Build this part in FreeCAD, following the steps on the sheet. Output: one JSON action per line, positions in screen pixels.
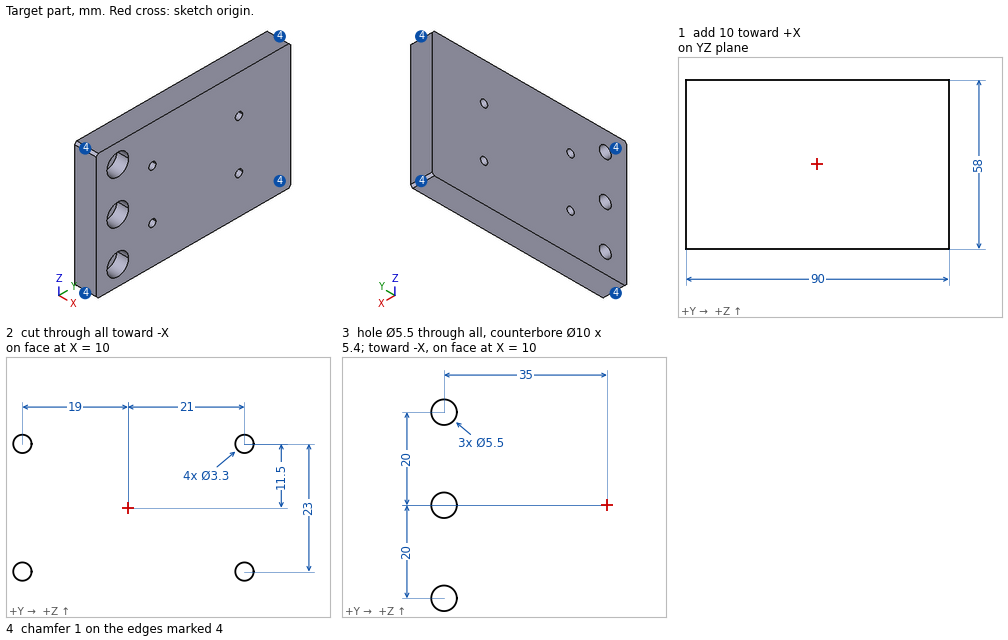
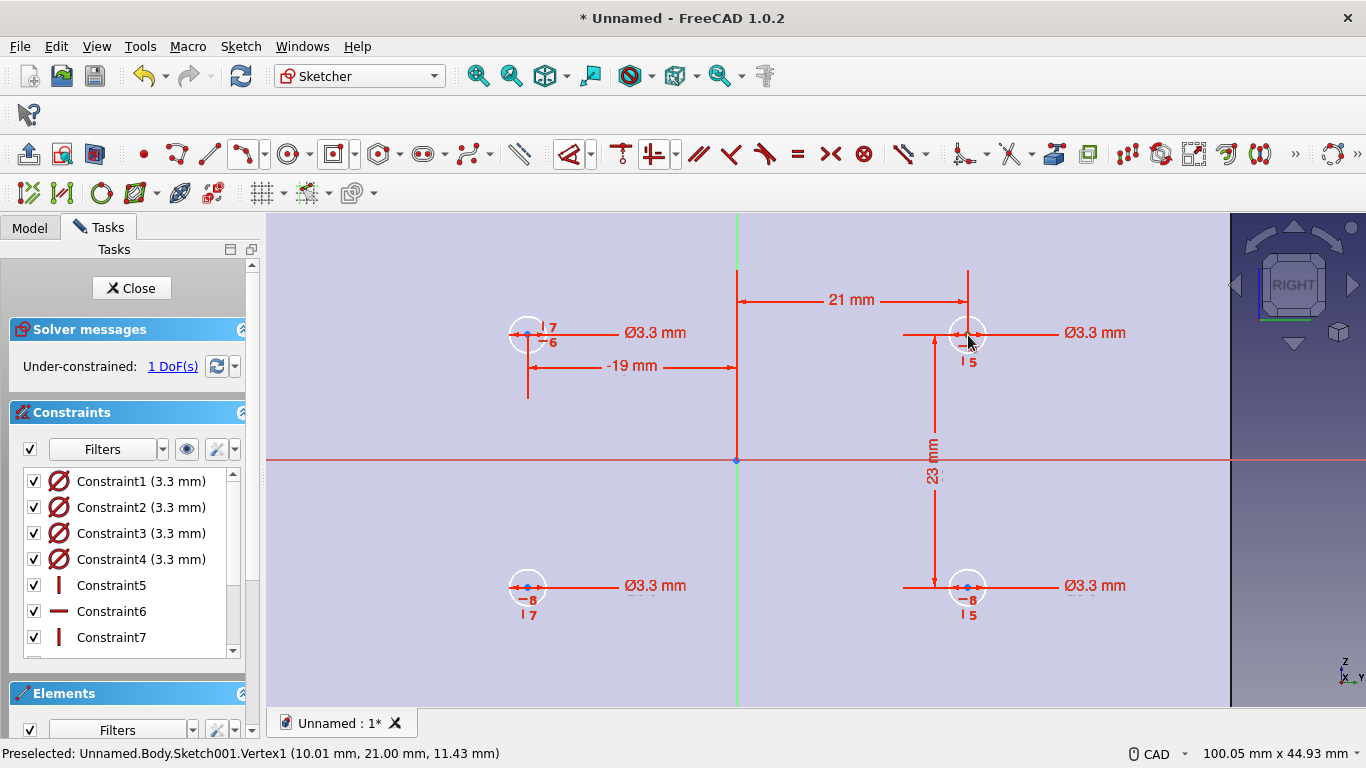
{"action": "key", "text": "i"}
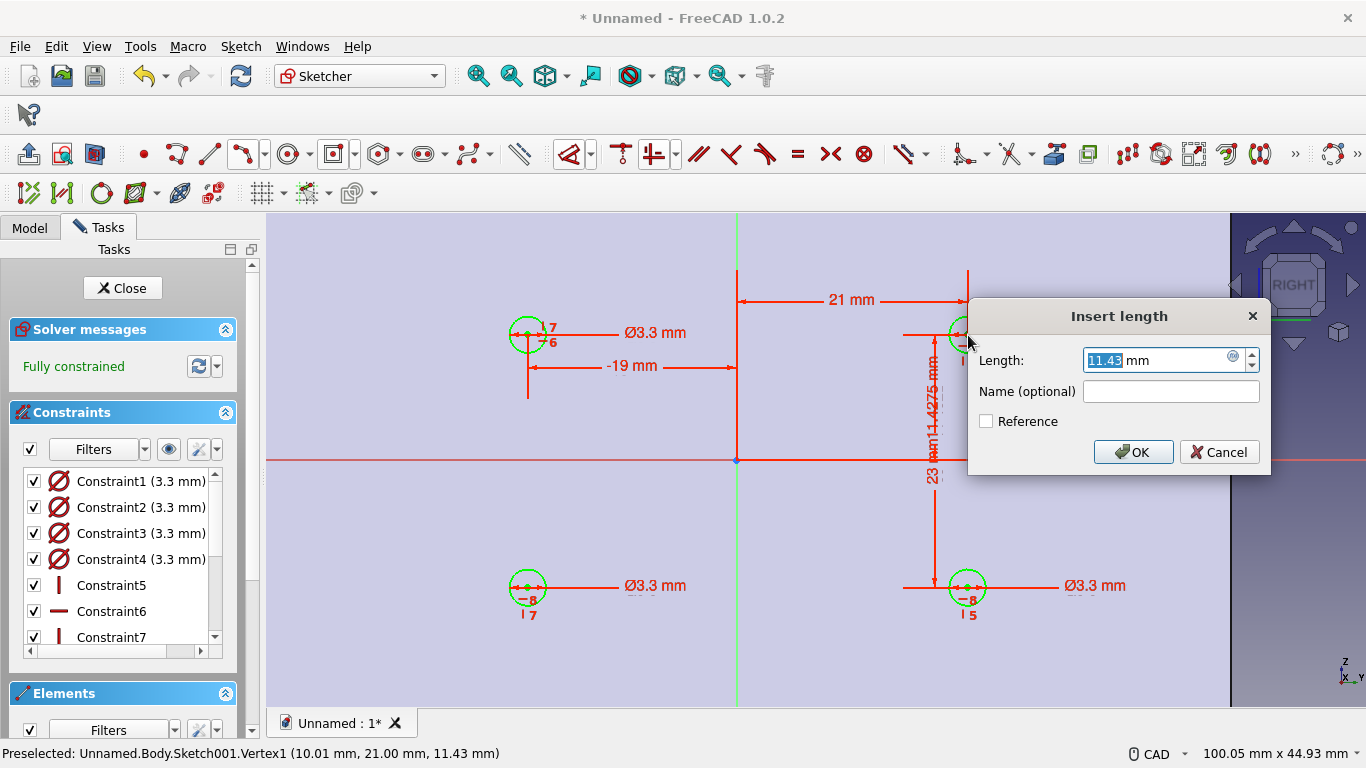
{"action": "type", "text": "11.5"}
{"action": "key", "text": "Return"}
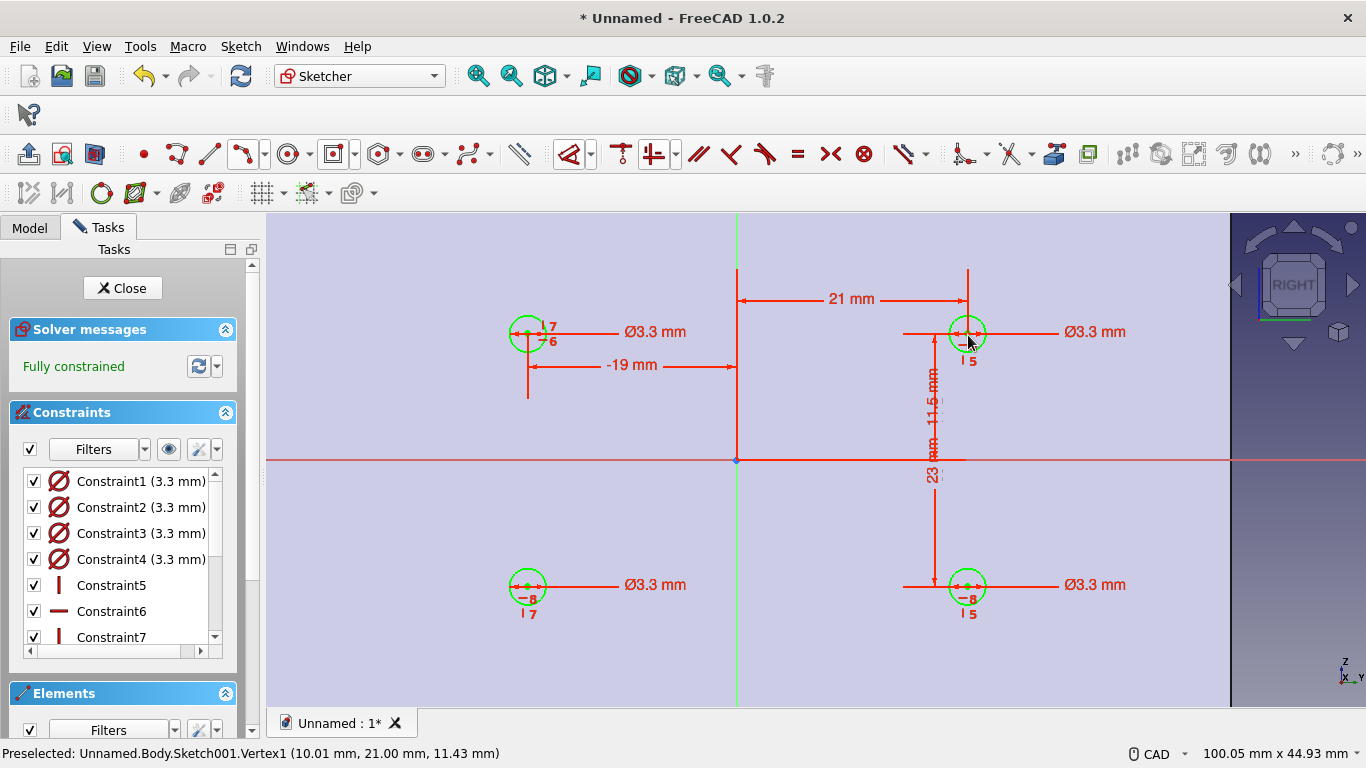
{"action": "left_click", "coordinate": [123, 288]}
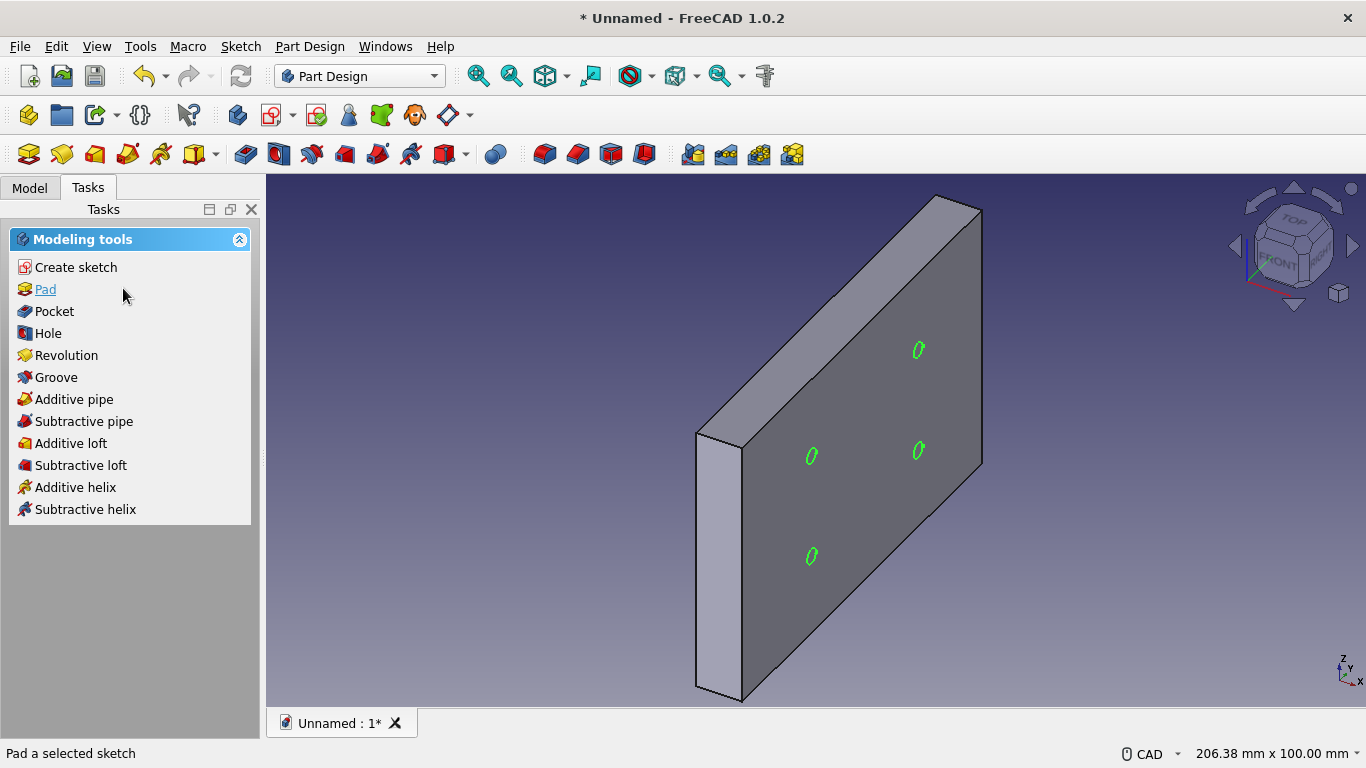
{"action": "left_click", "coordinate": [246, 154]}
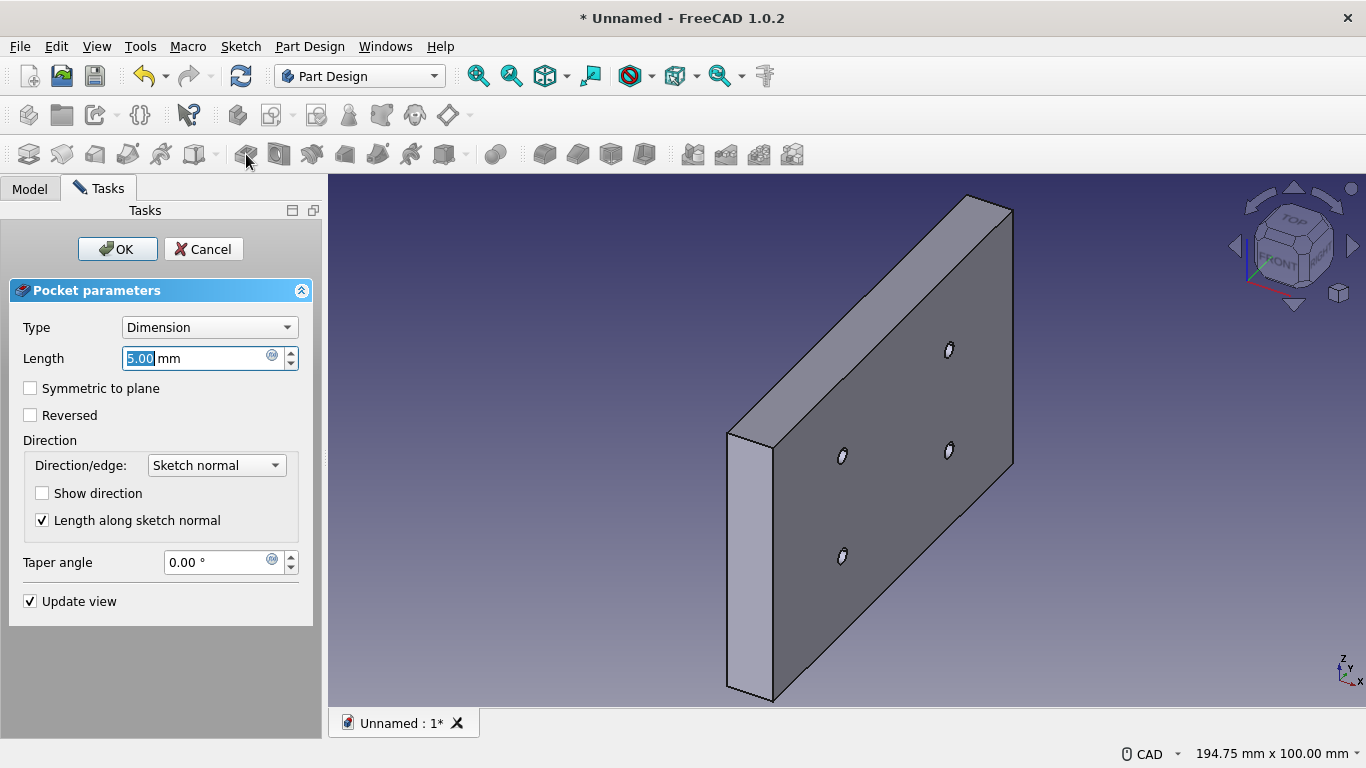
{"action": "left_click", "coordinate": [210, 328]}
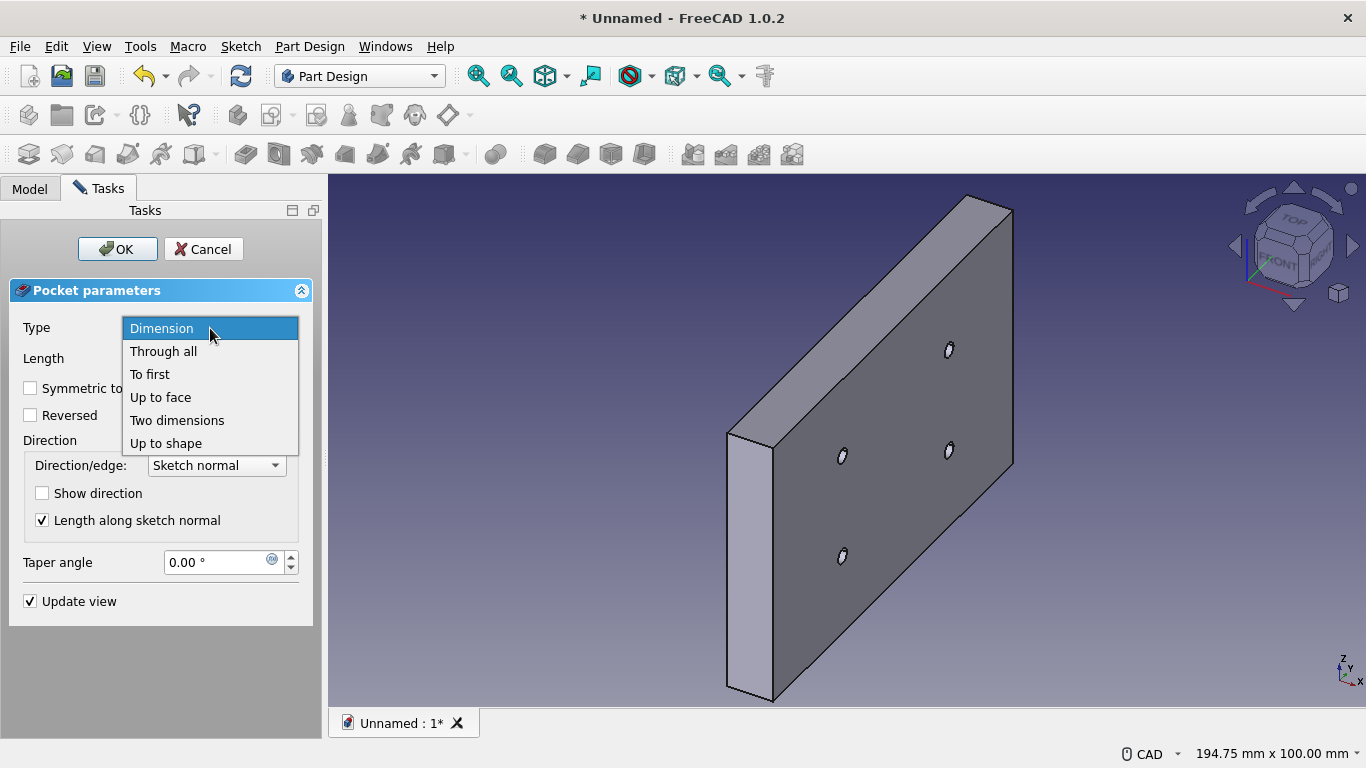
{"action": "left_click", "coordinate": [208, 352]}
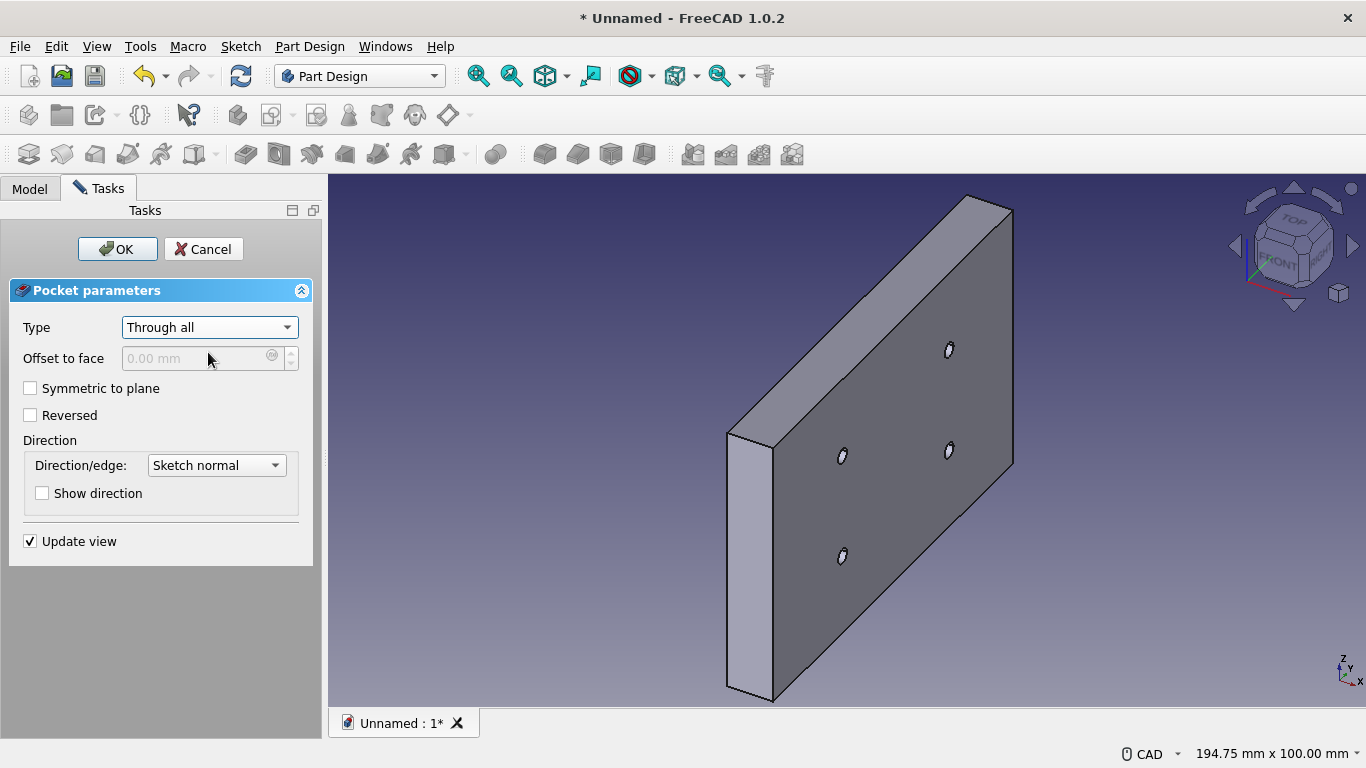
{"action": "left_click", "coordinate": [118, 249]}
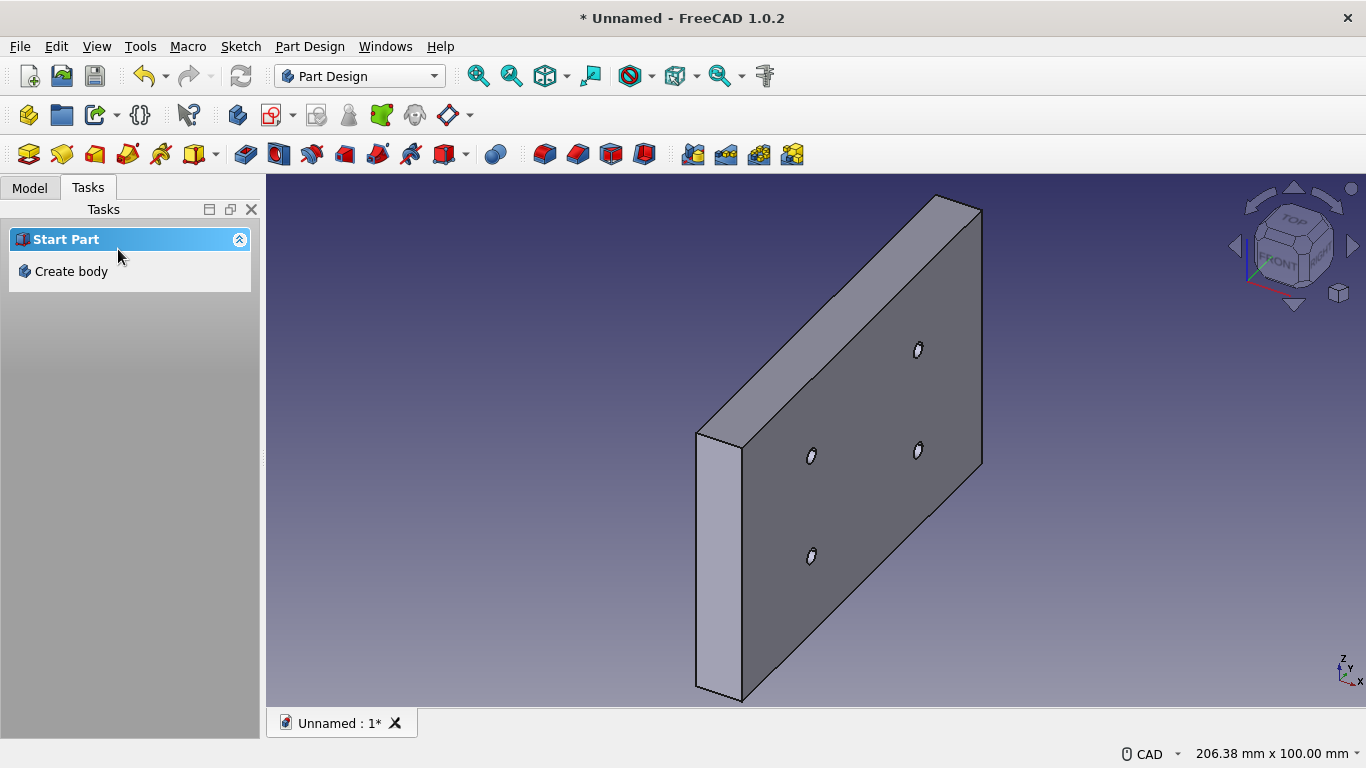
{"action": "left_click", "coordinate": [862, 455]}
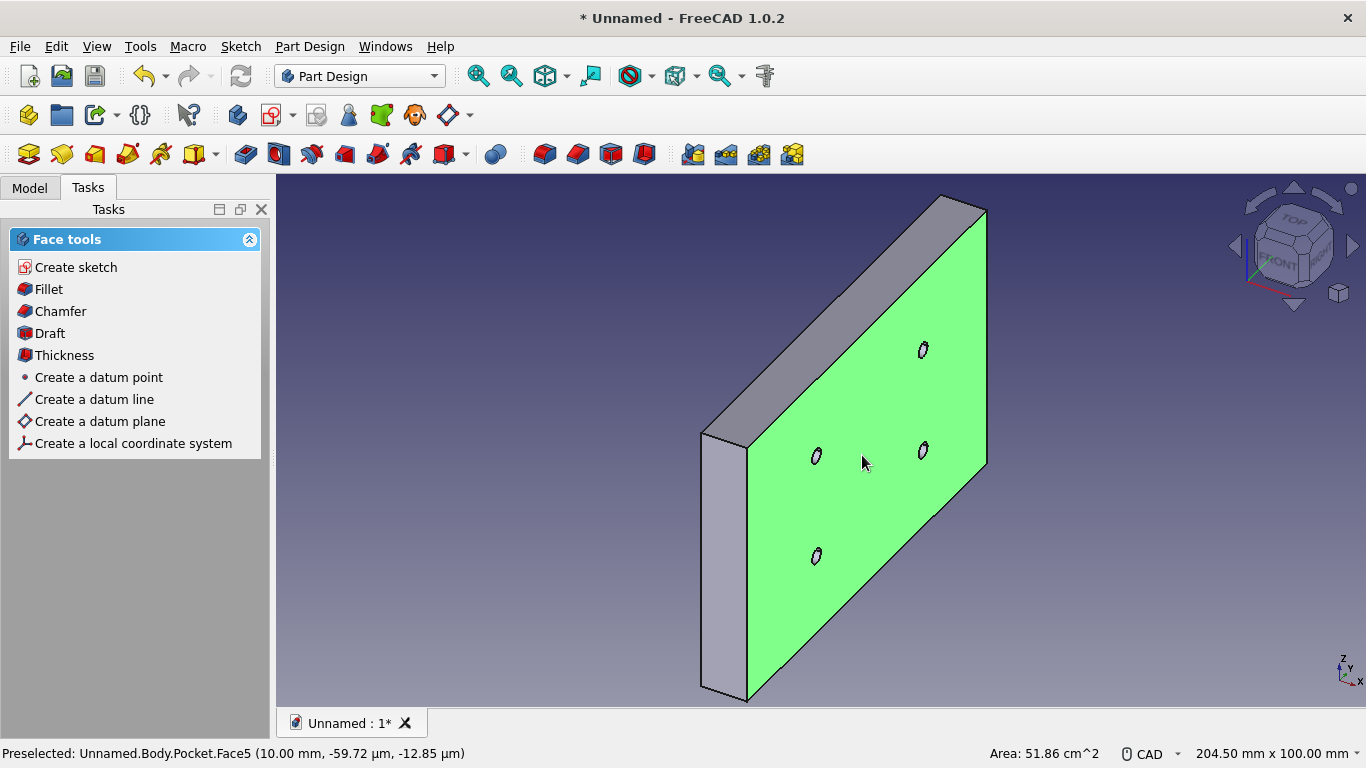
{"action": "left_click", "coordinate": [270, 116]}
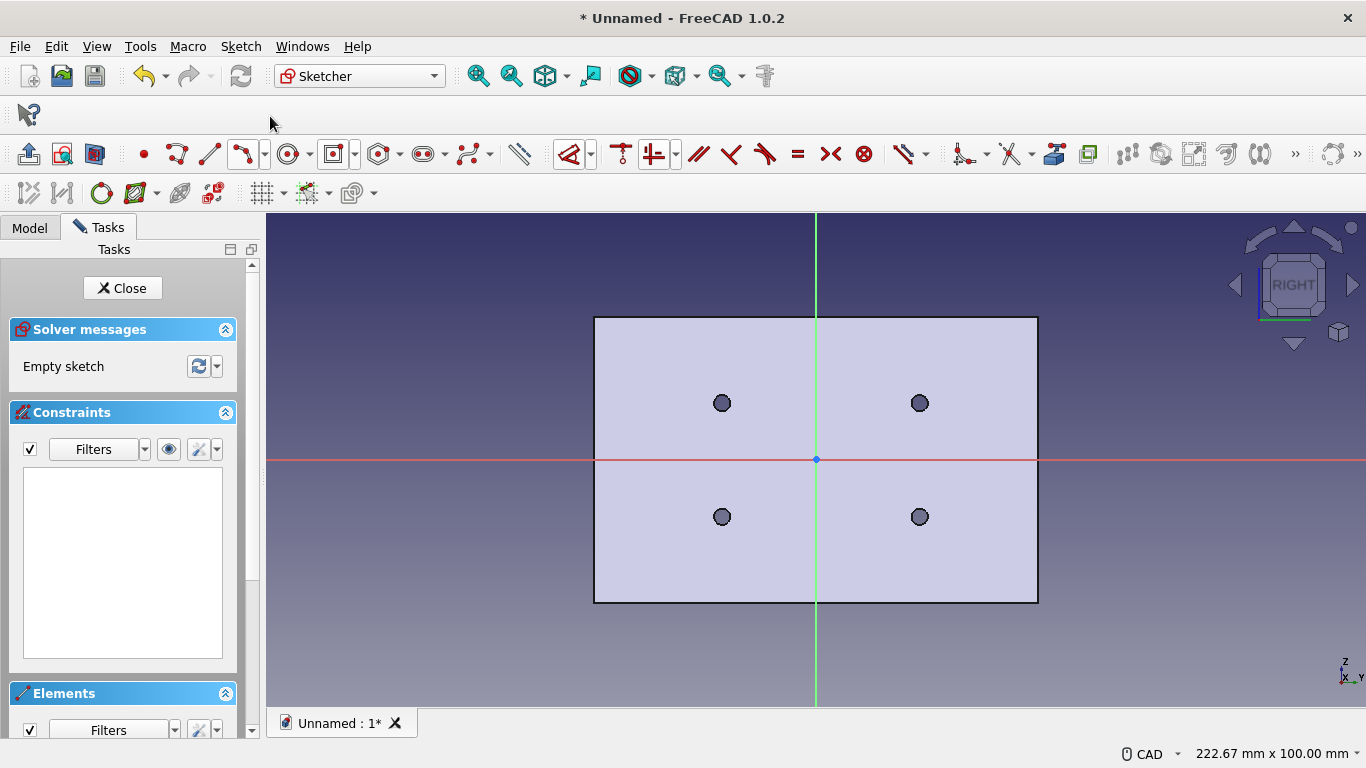
{"action": "scroll", "coordinate": [672, 460], "scroll_direction": "up", "scroll_amount": 2}